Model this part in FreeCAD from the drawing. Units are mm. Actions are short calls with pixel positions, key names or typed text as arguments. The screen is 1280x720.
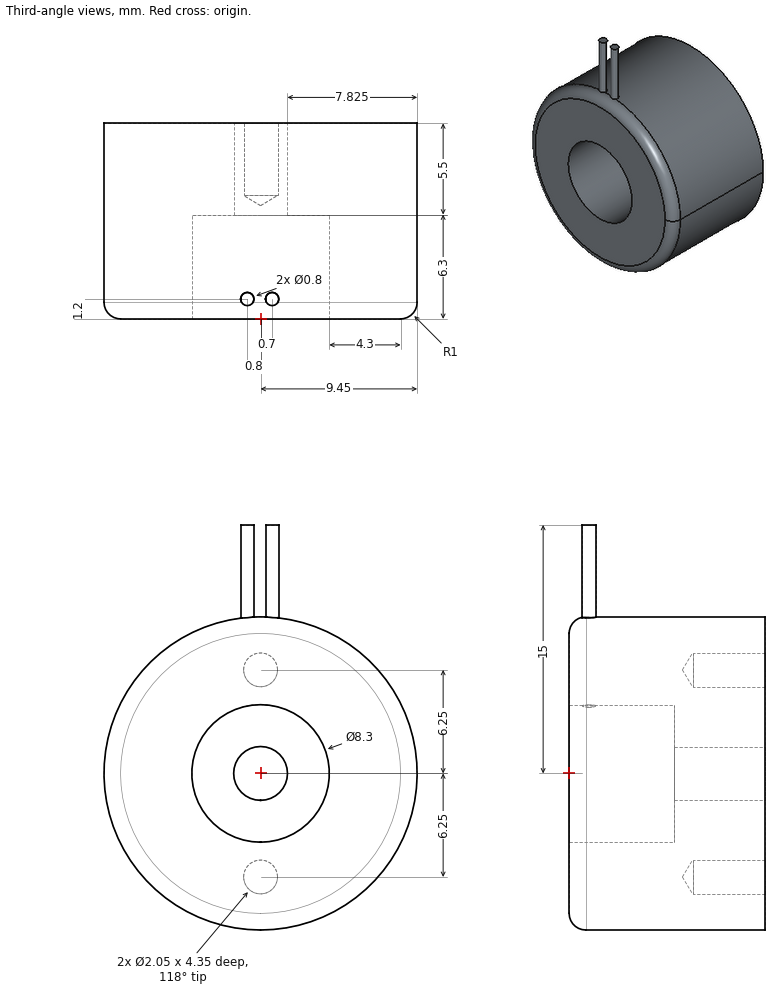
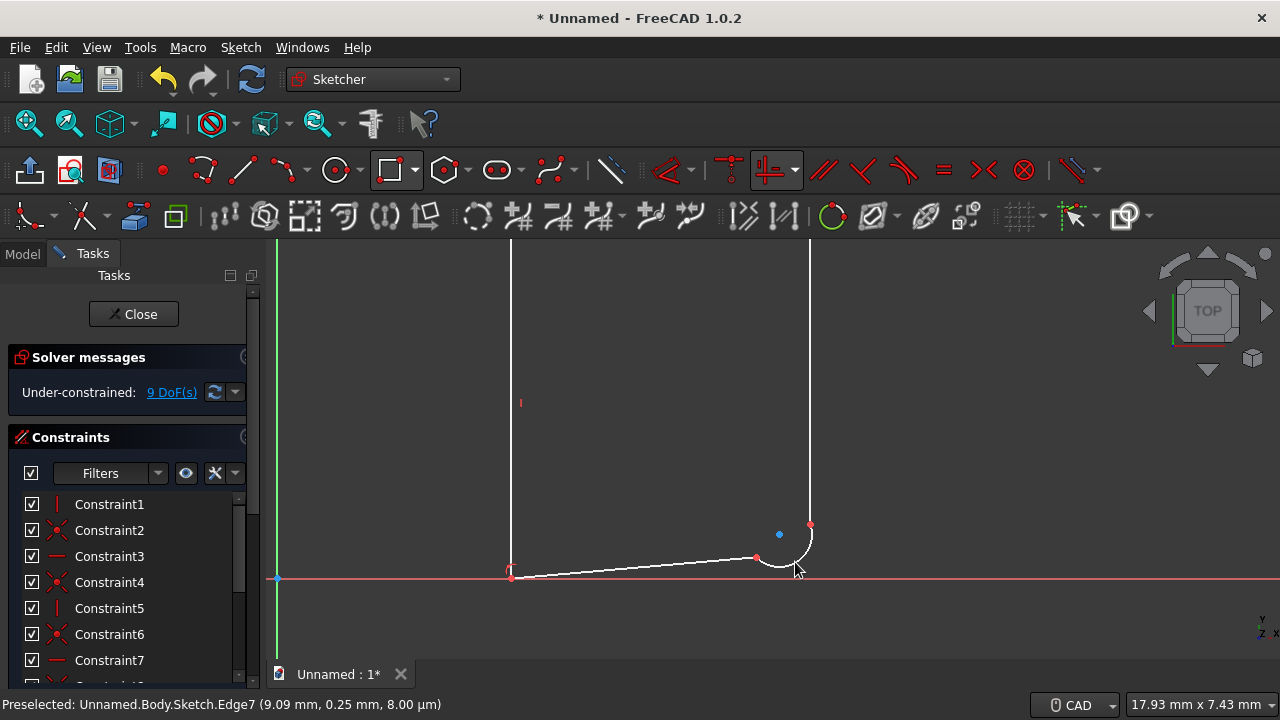
click(810, 341)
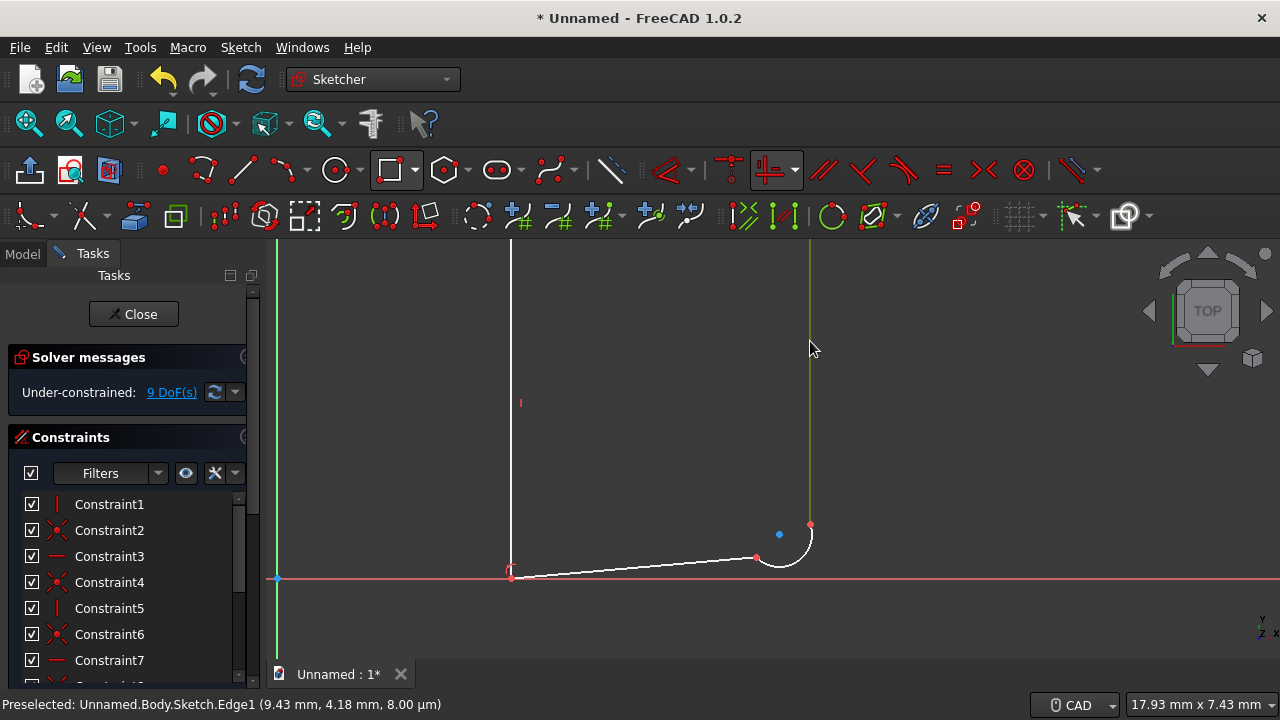
click(780, 567)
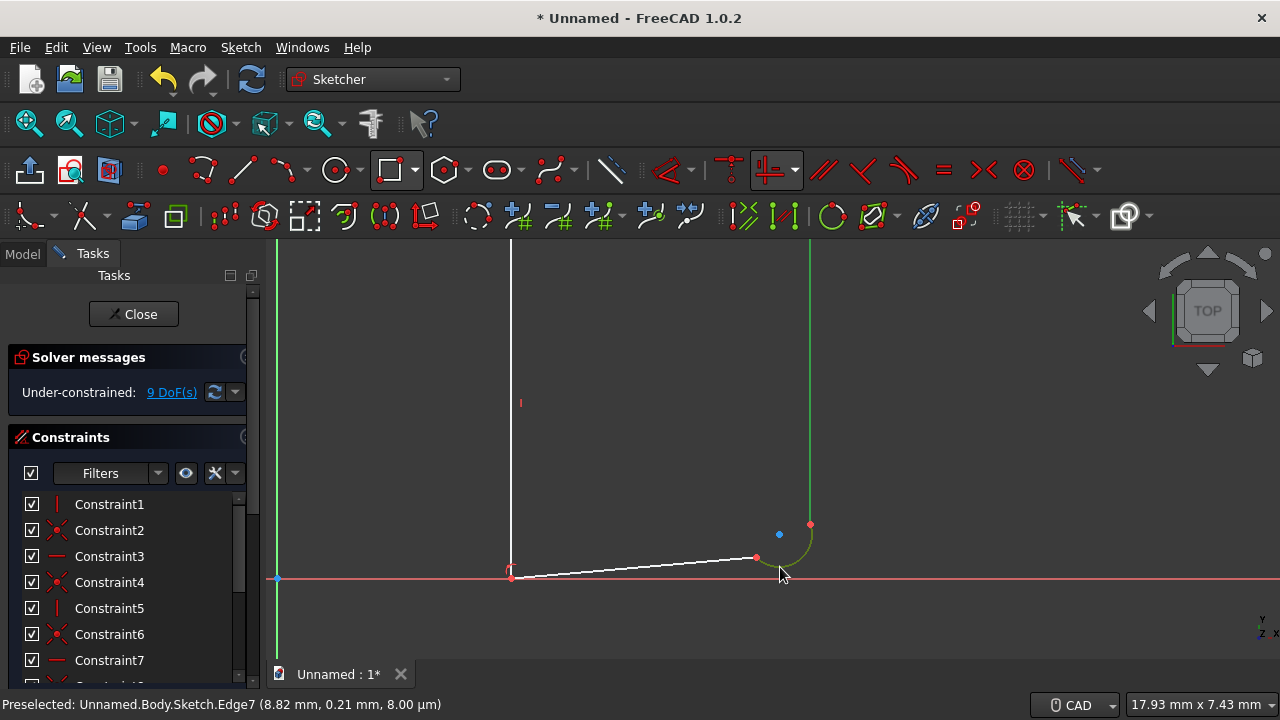
key(t)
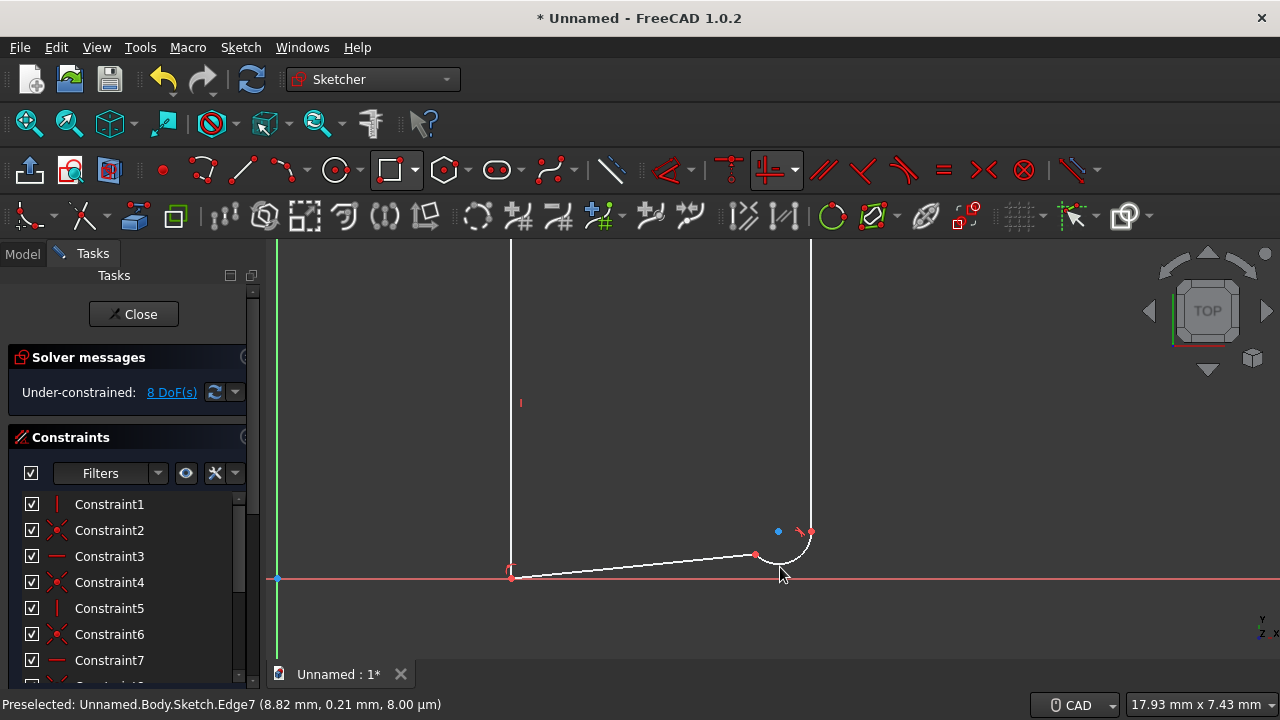
click(682, 562)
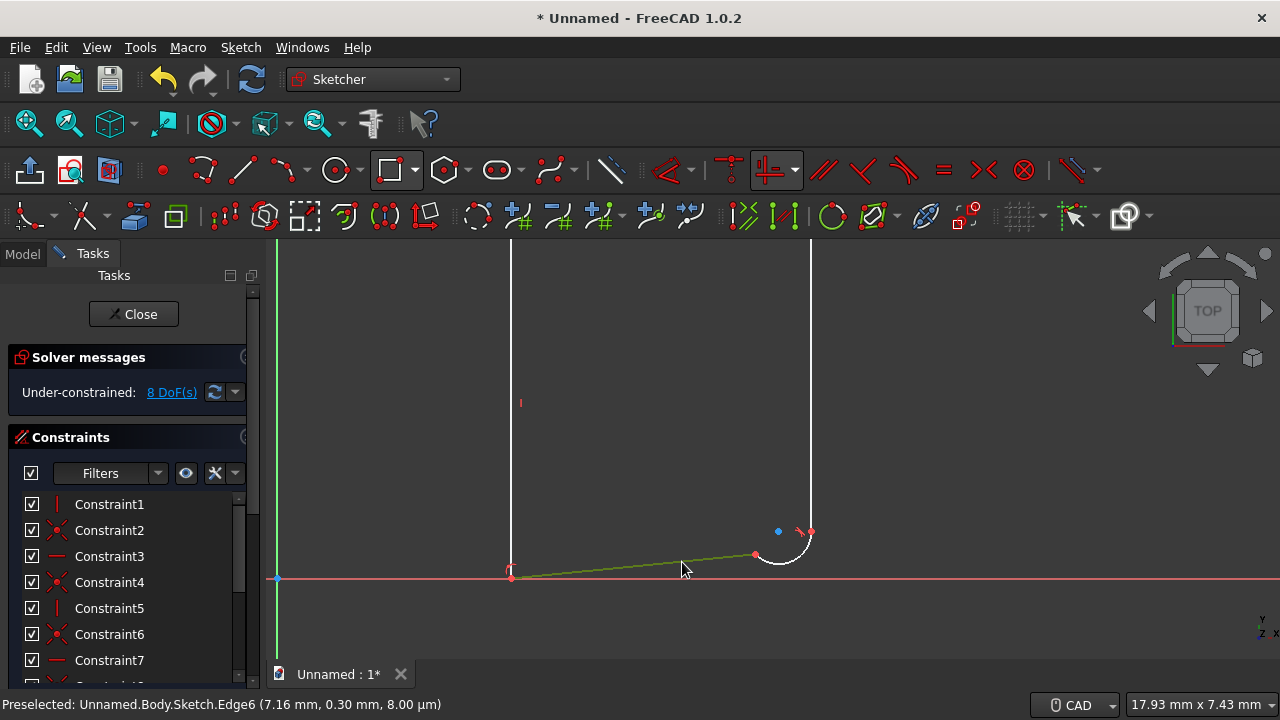
click(776, 564)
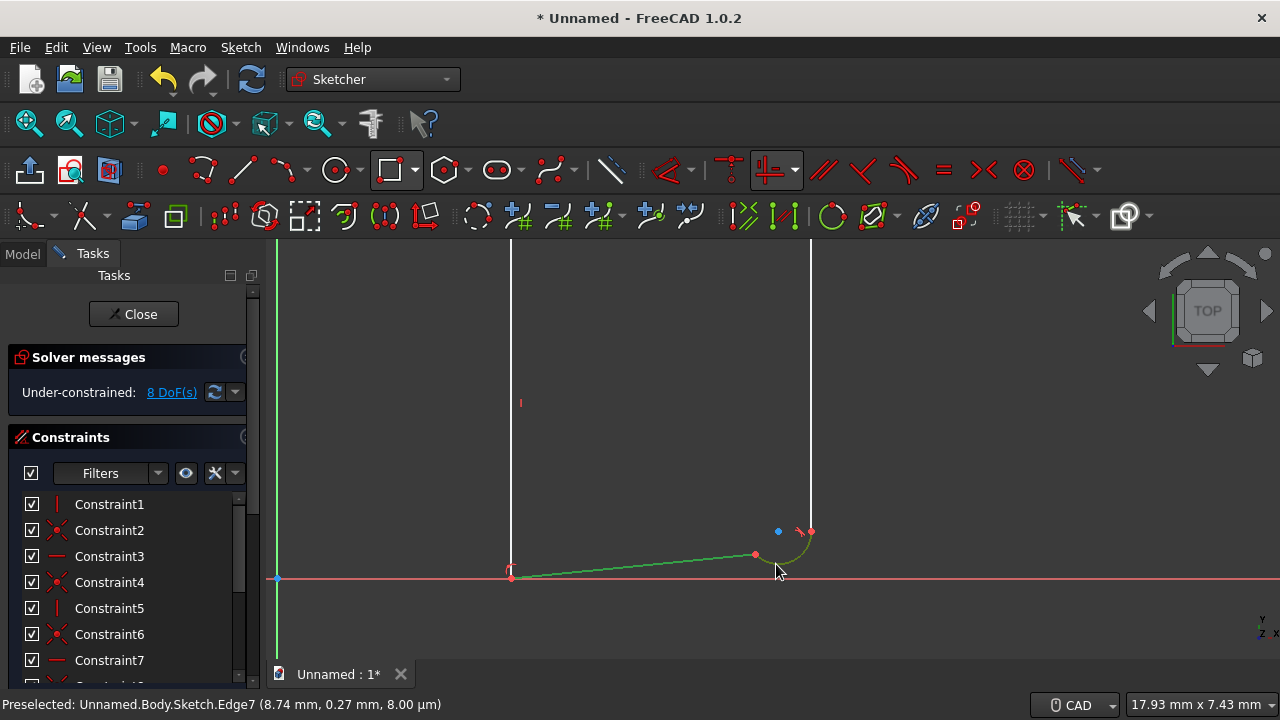
click(904, 170)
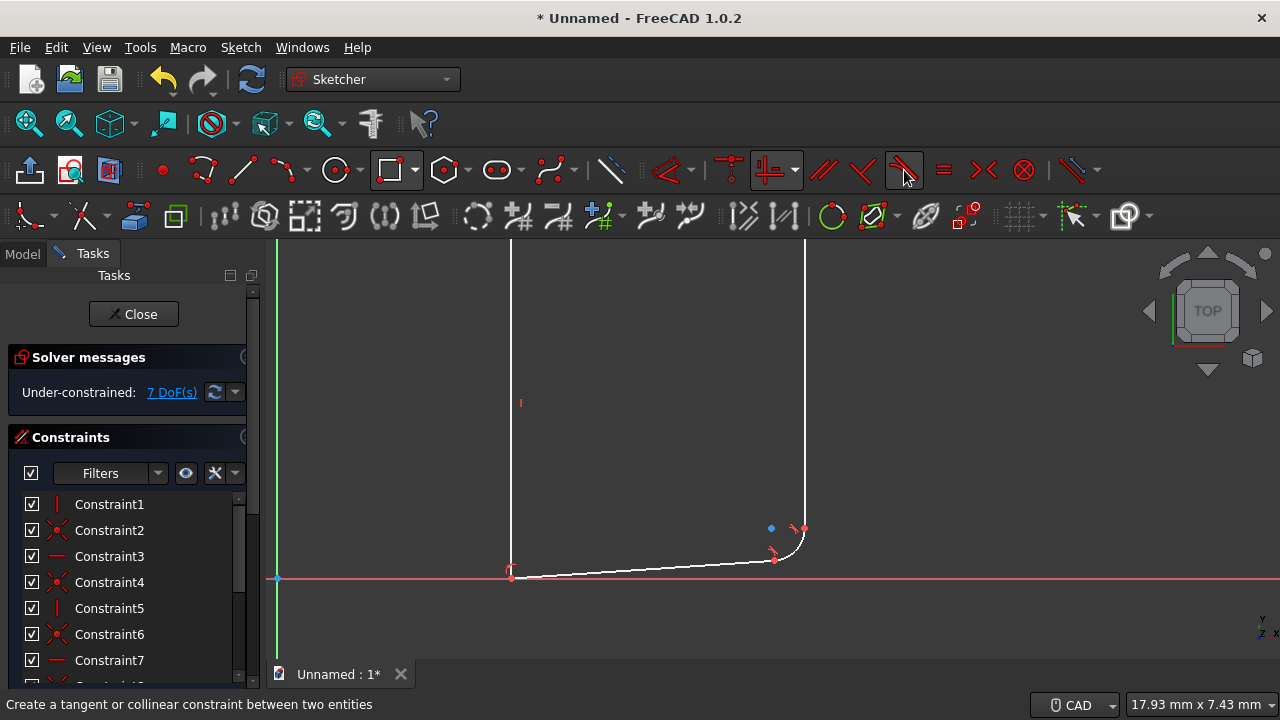
click(695, 566)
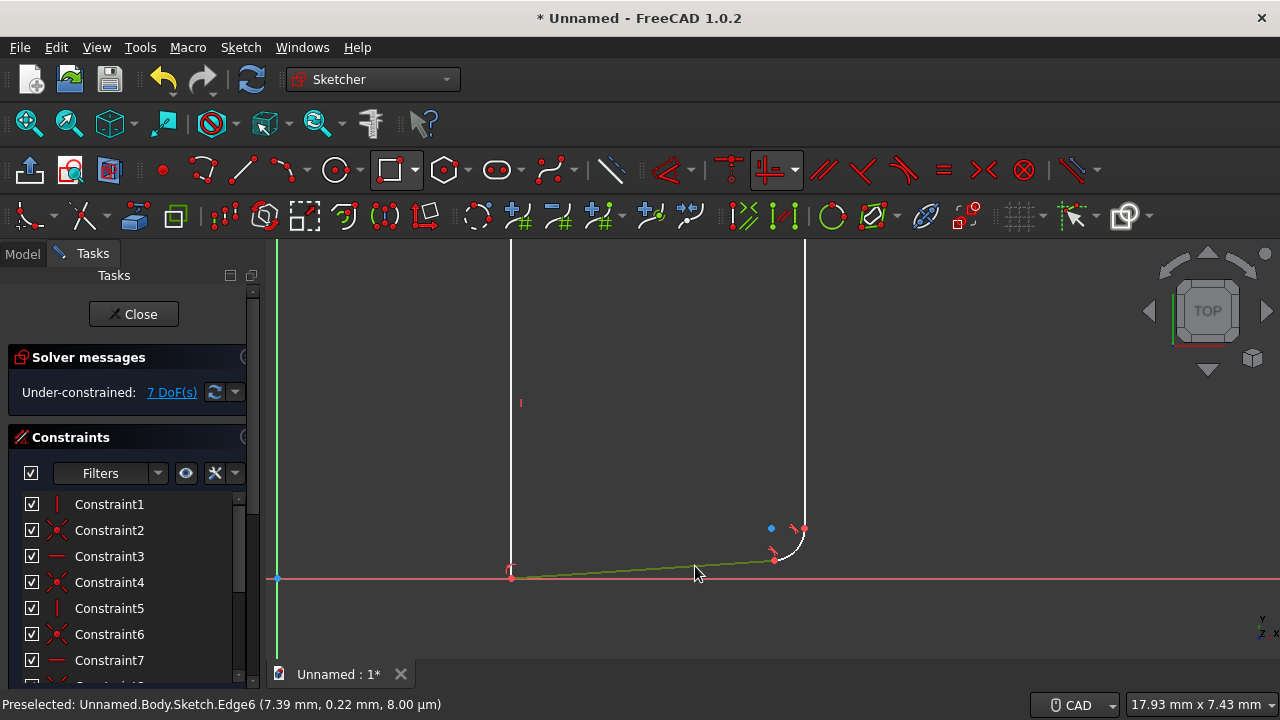
key(h)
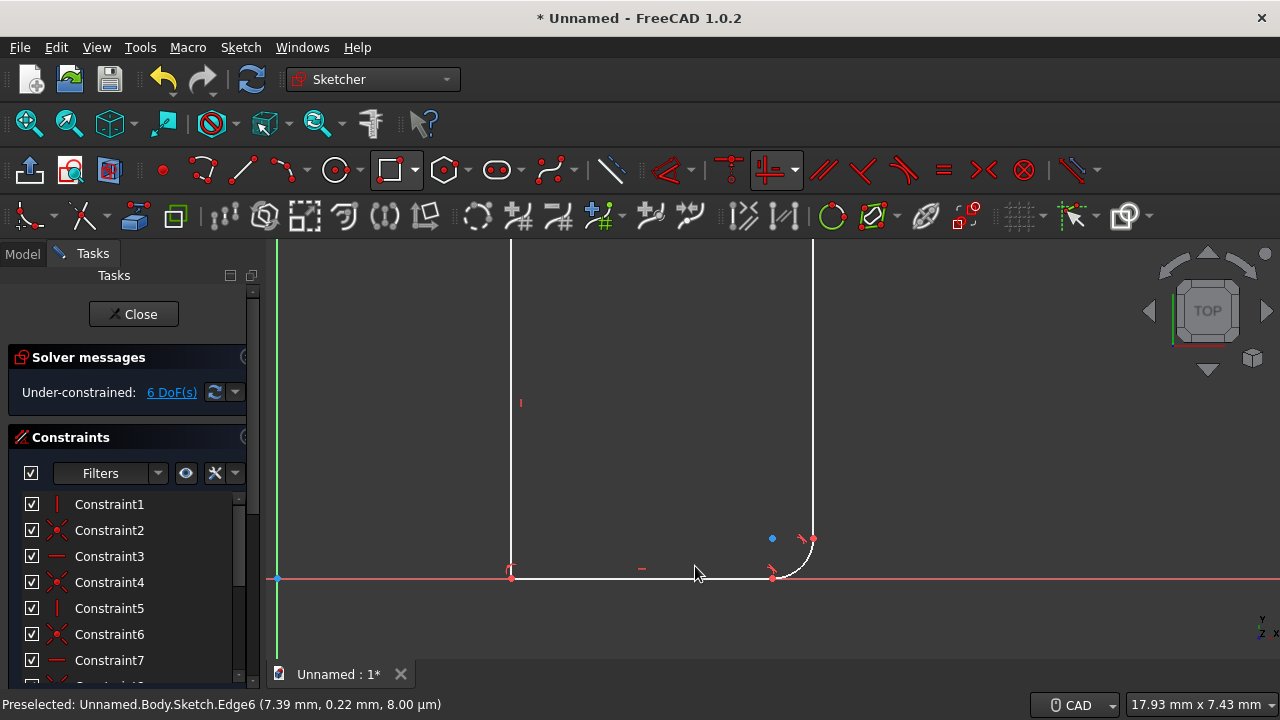
click(666, 170)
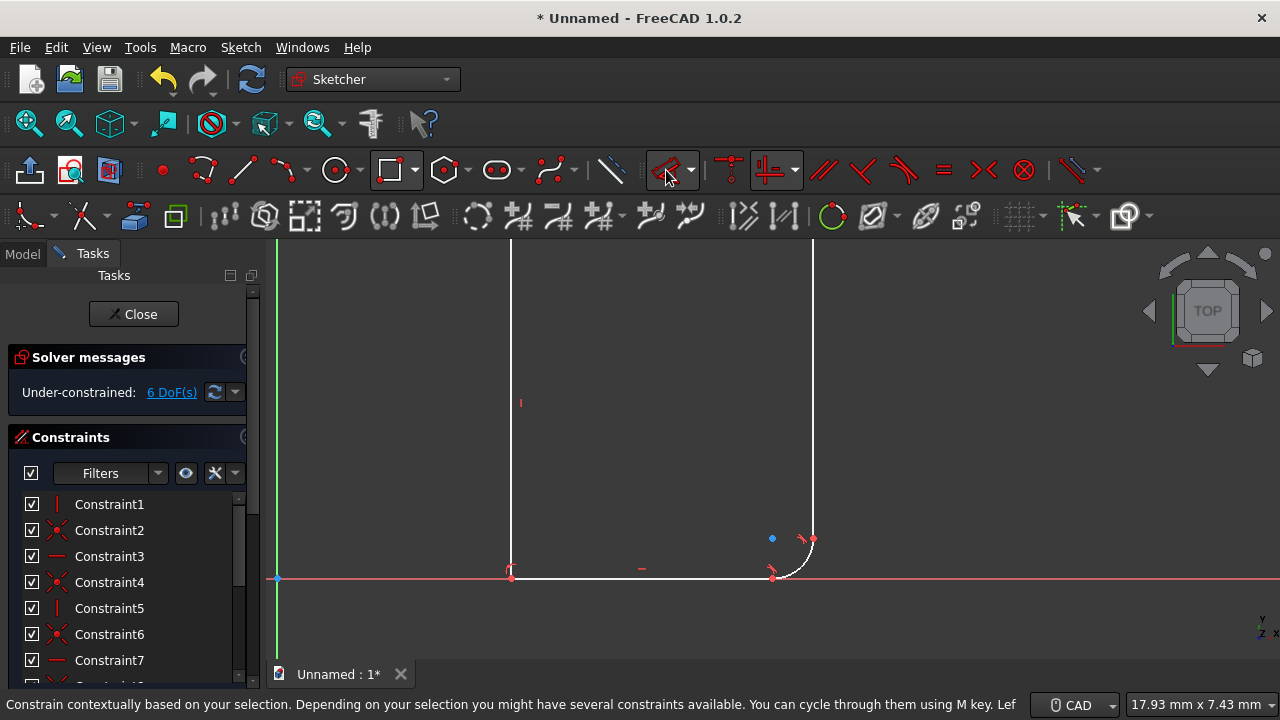
click(809, 556)
click(814, 597)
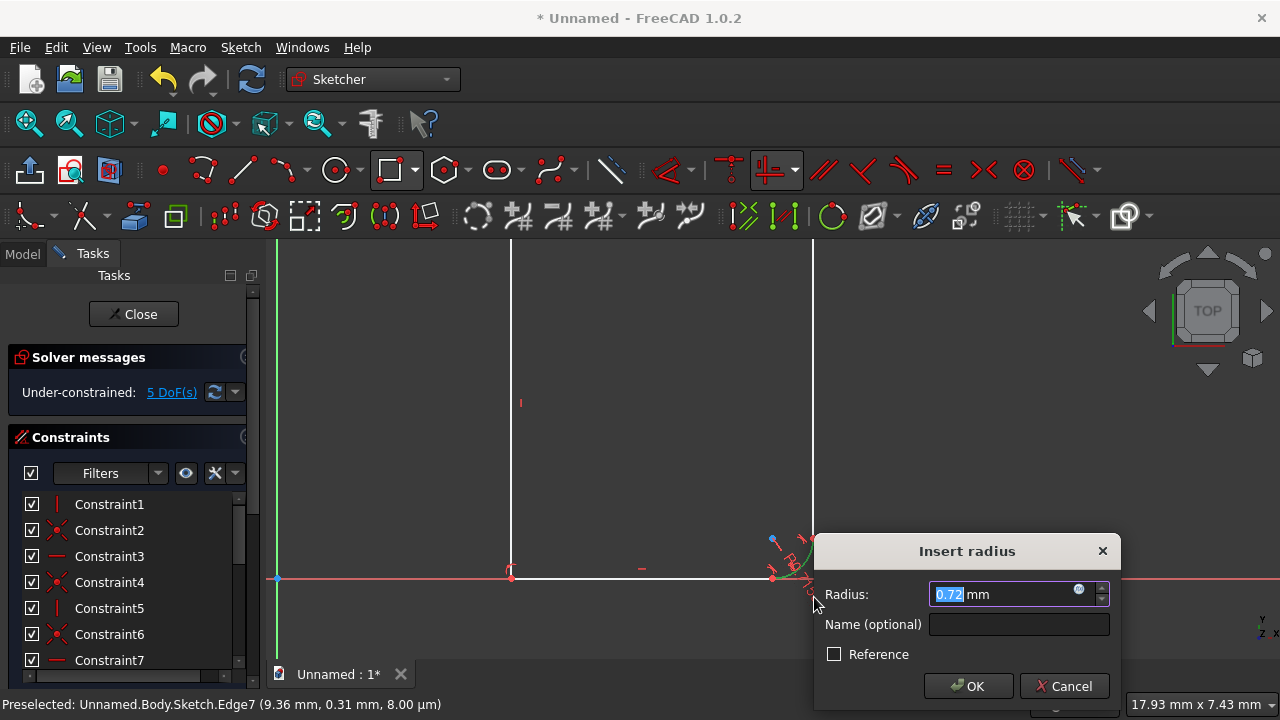
text(1)
key(Return)